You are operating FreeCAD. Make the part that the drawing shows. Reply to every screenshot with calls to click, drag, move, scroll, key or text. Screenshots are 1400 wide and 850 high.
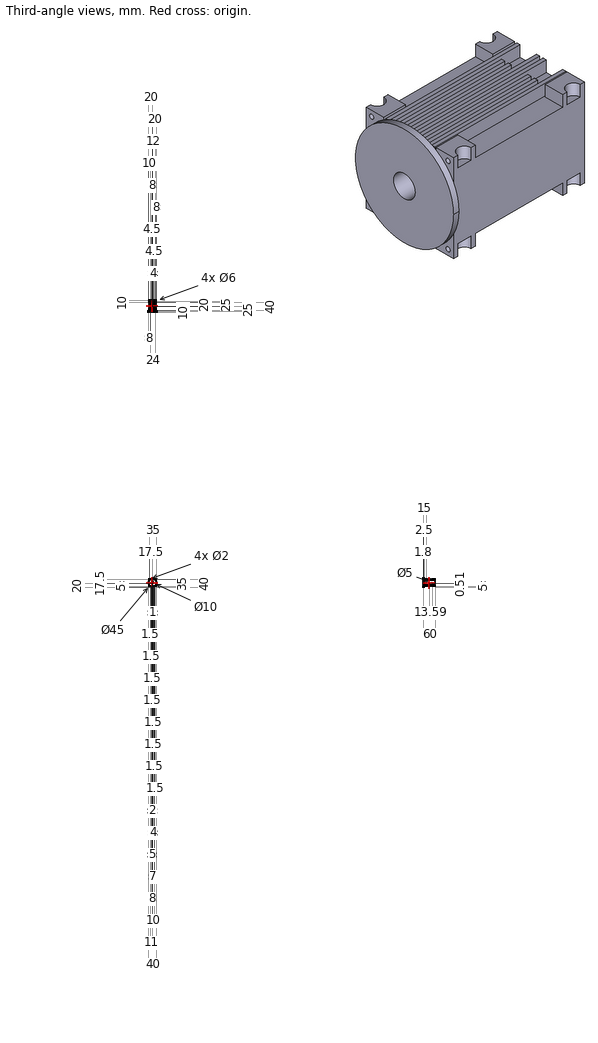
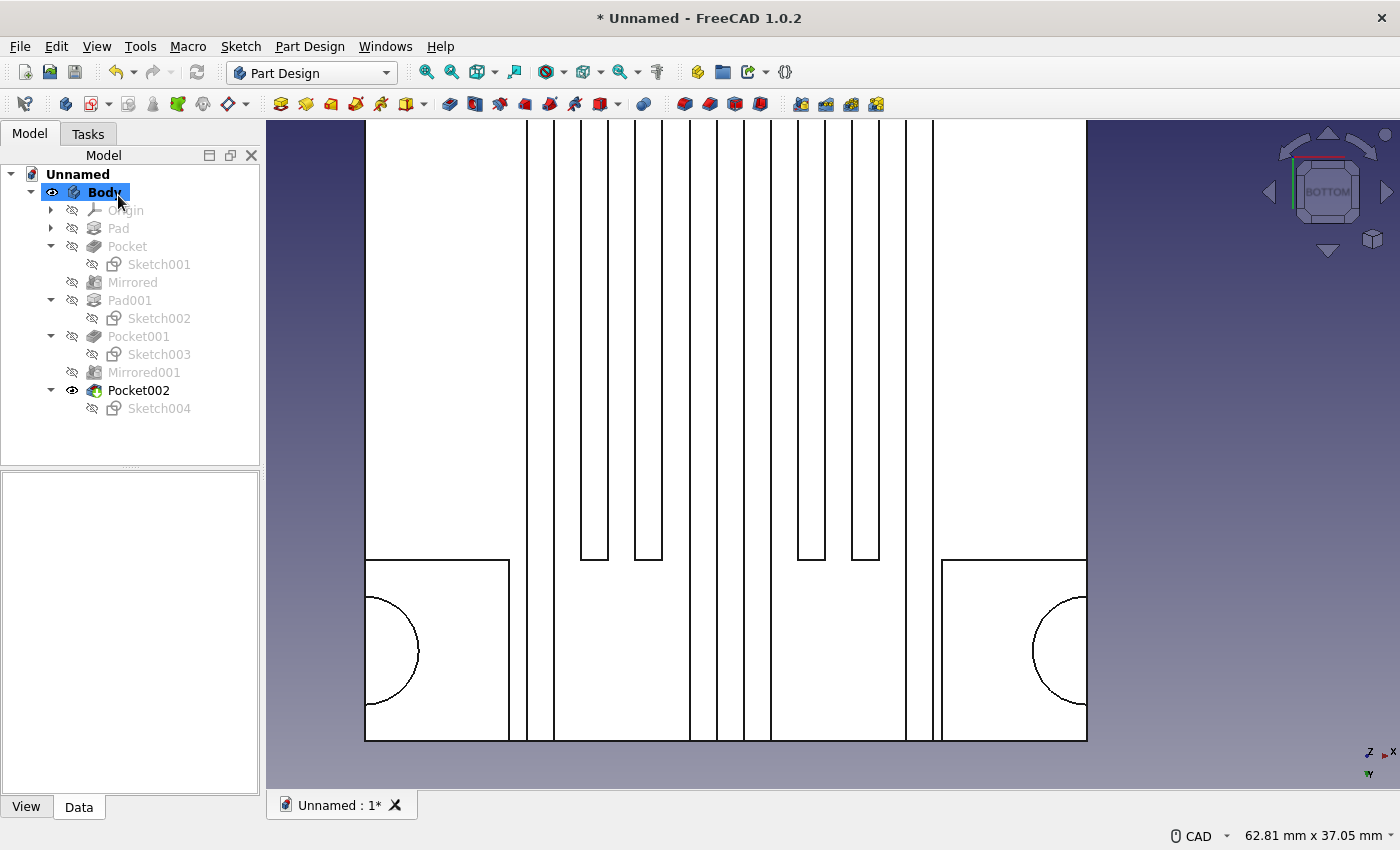
click(427, 72)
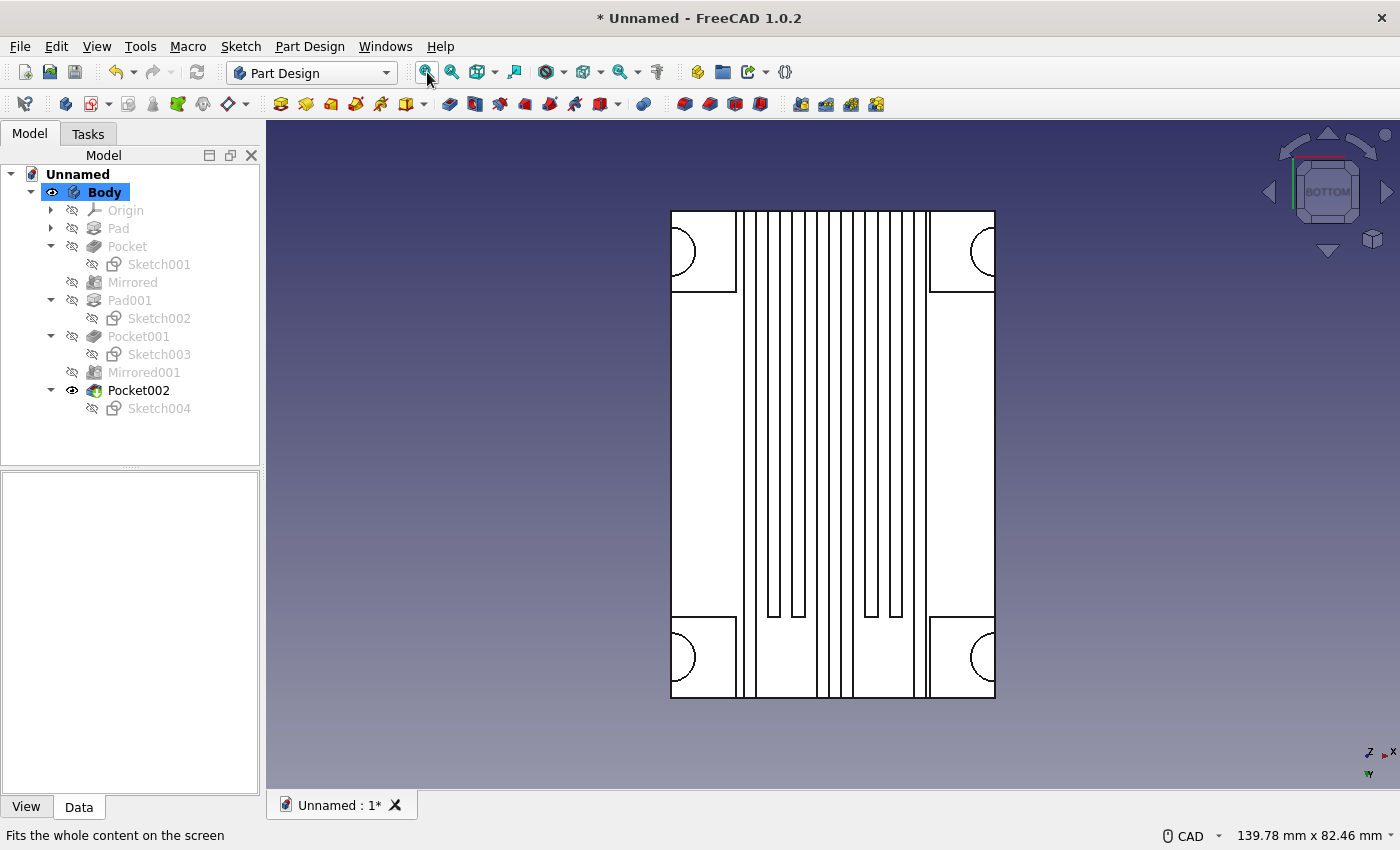
click(117, 390)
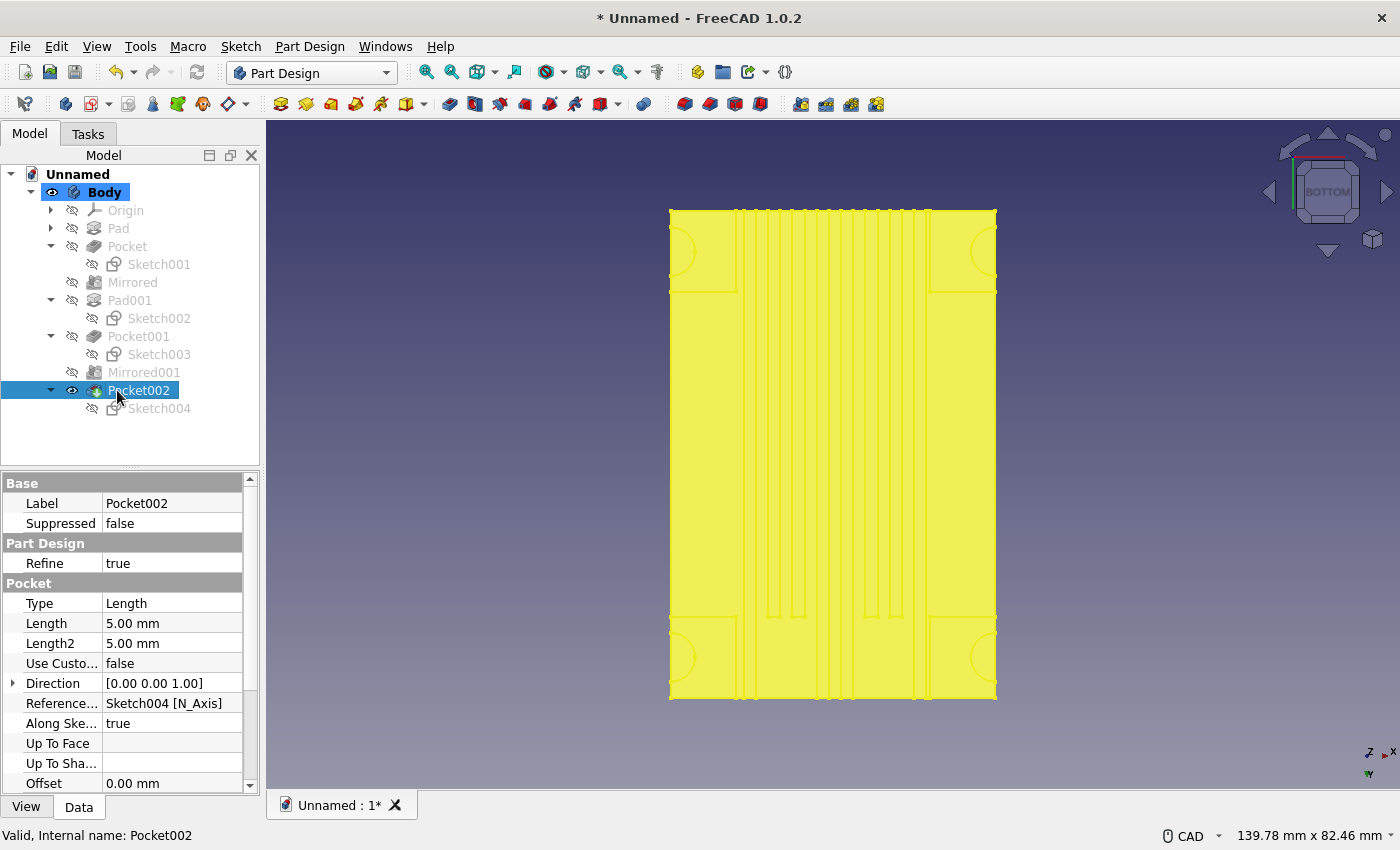
click(801, 104)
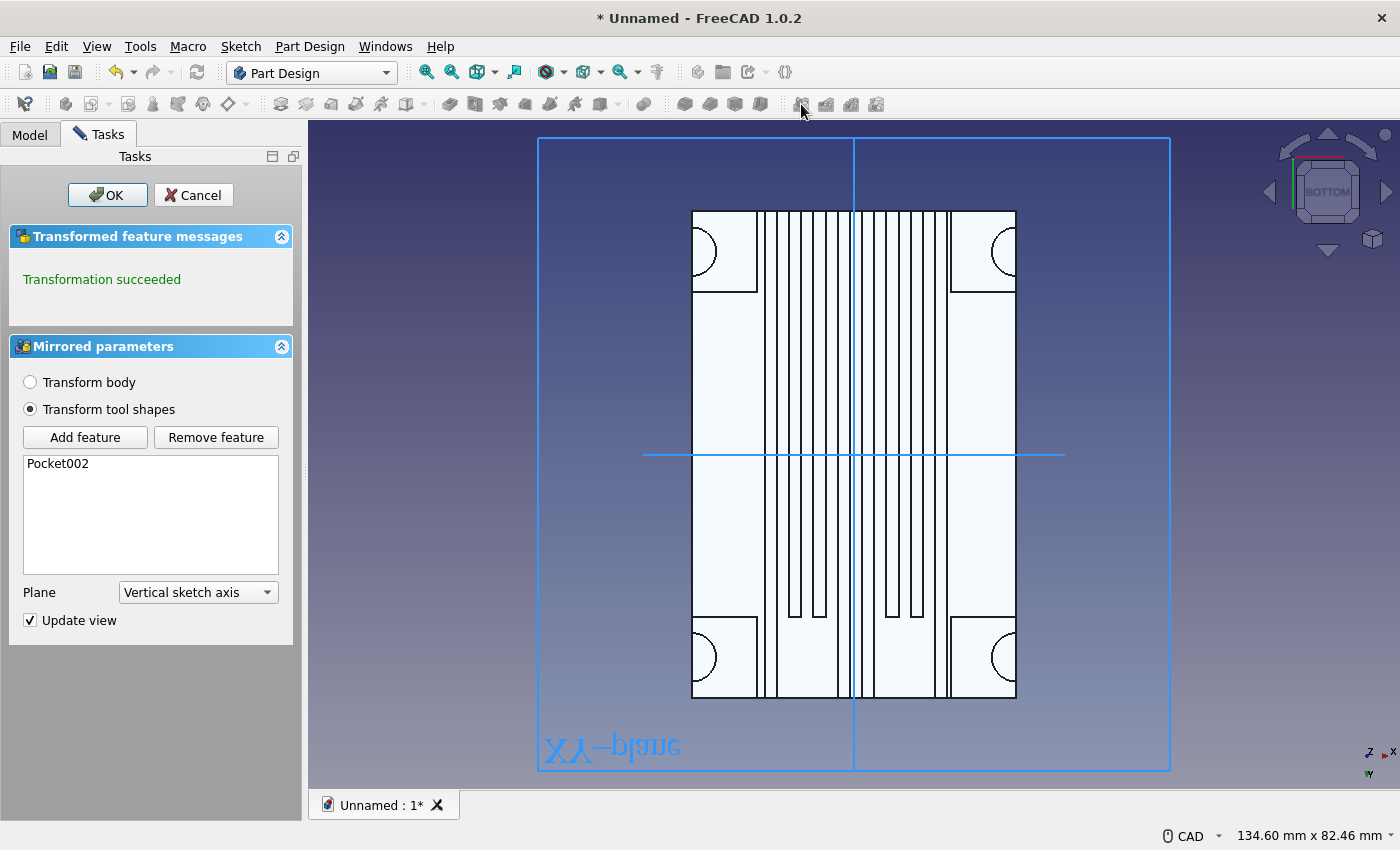
click(199, 592)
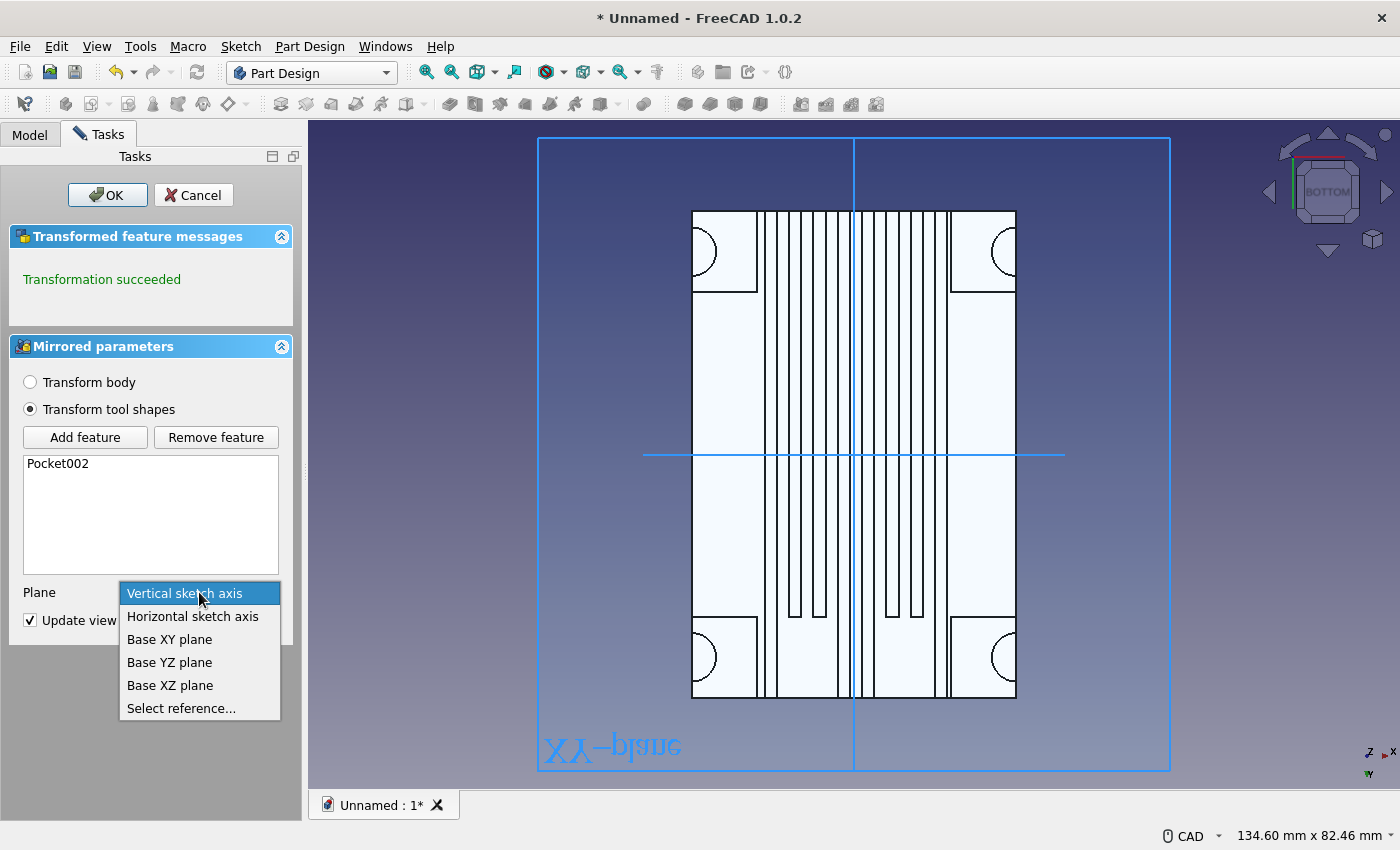
click(198, 640)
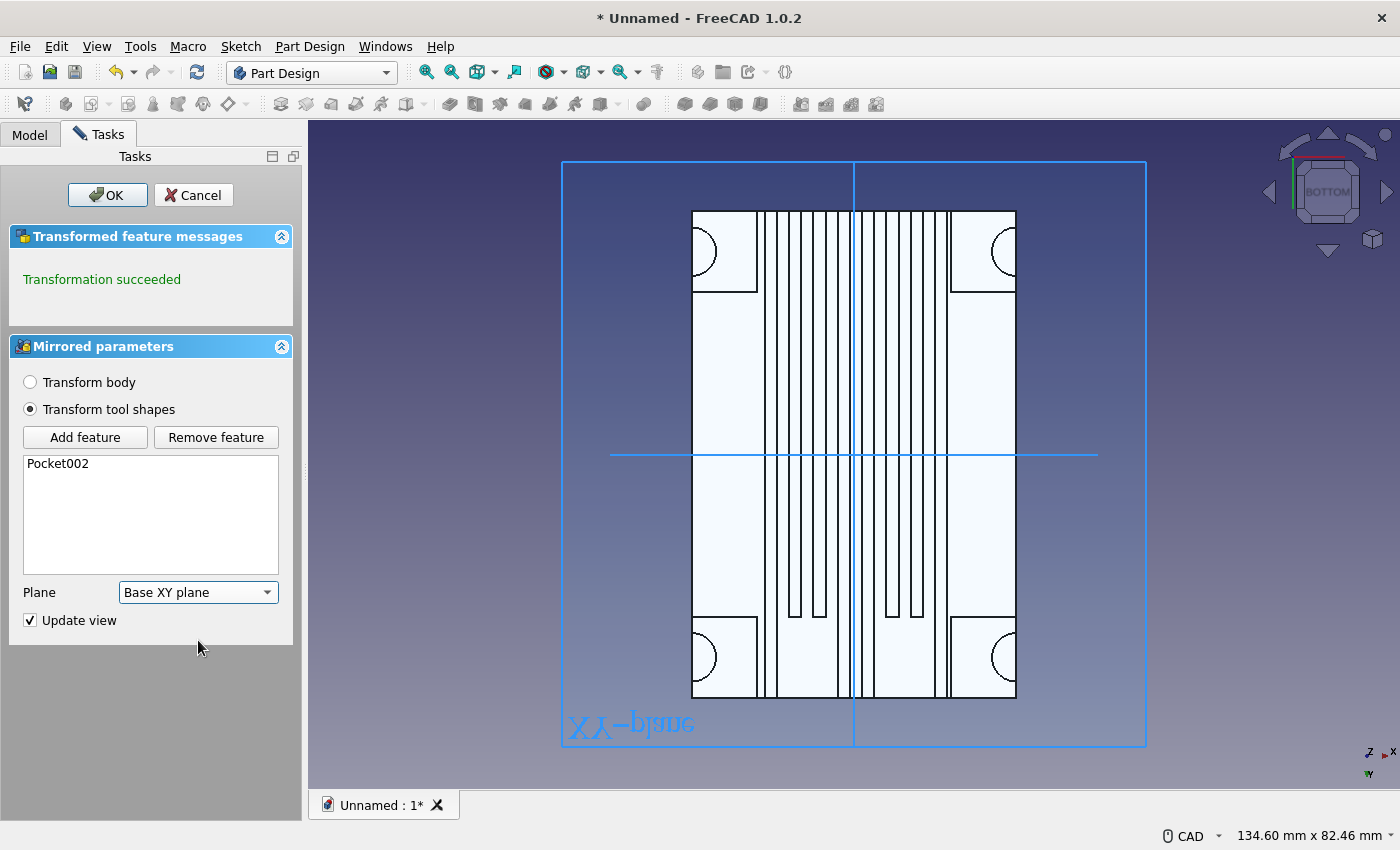
click(108, 195)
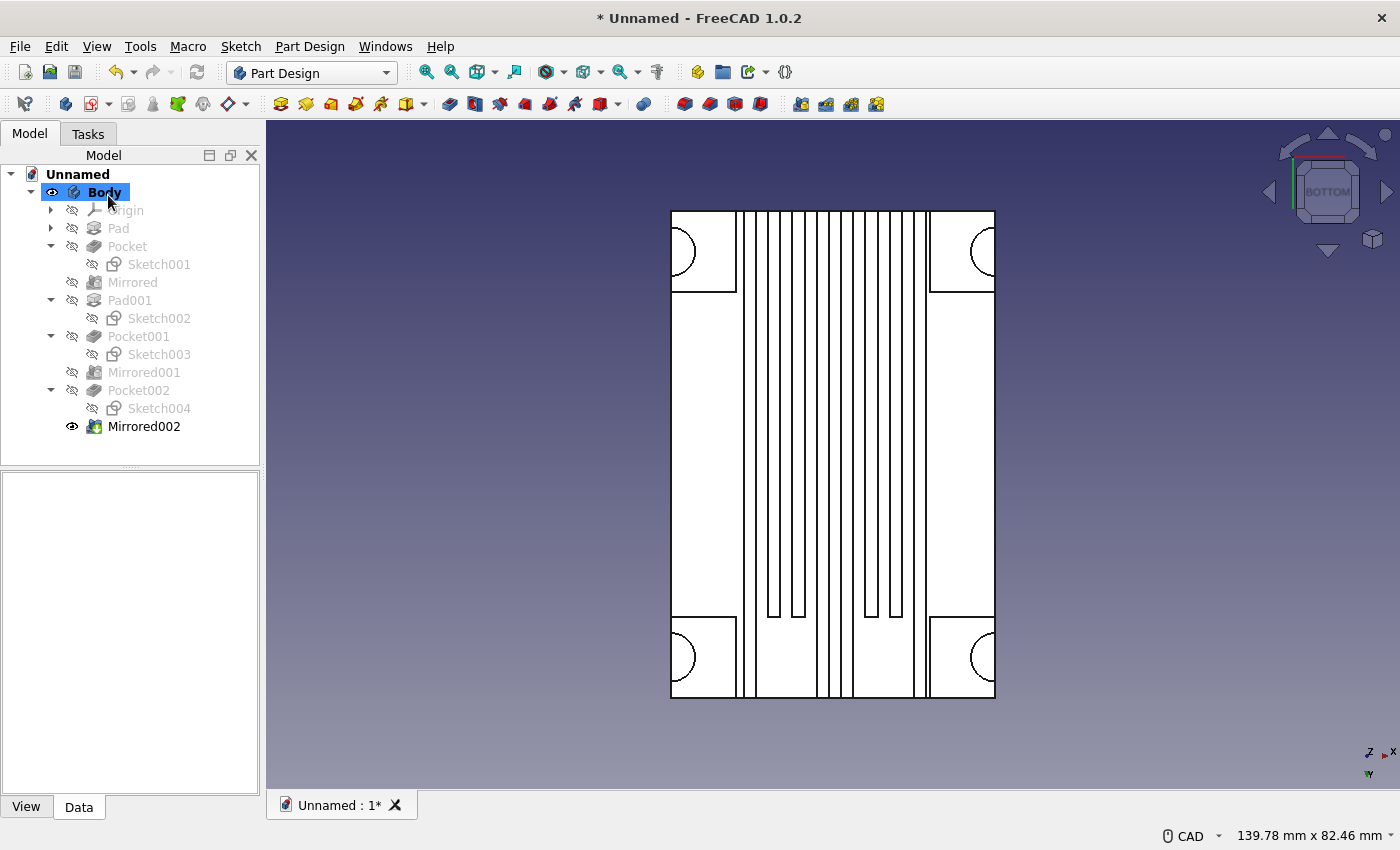
key(0)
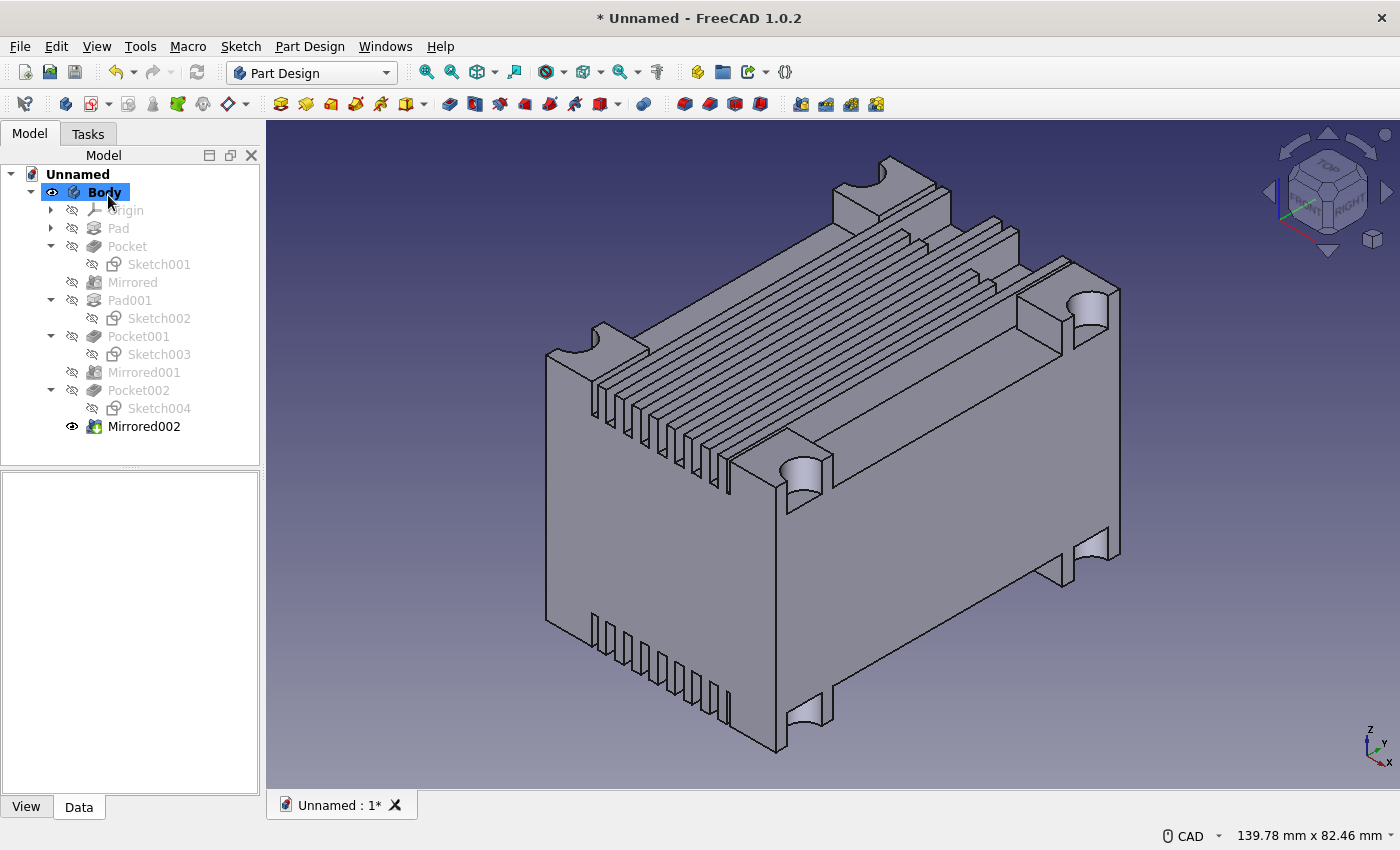
click(661, 553)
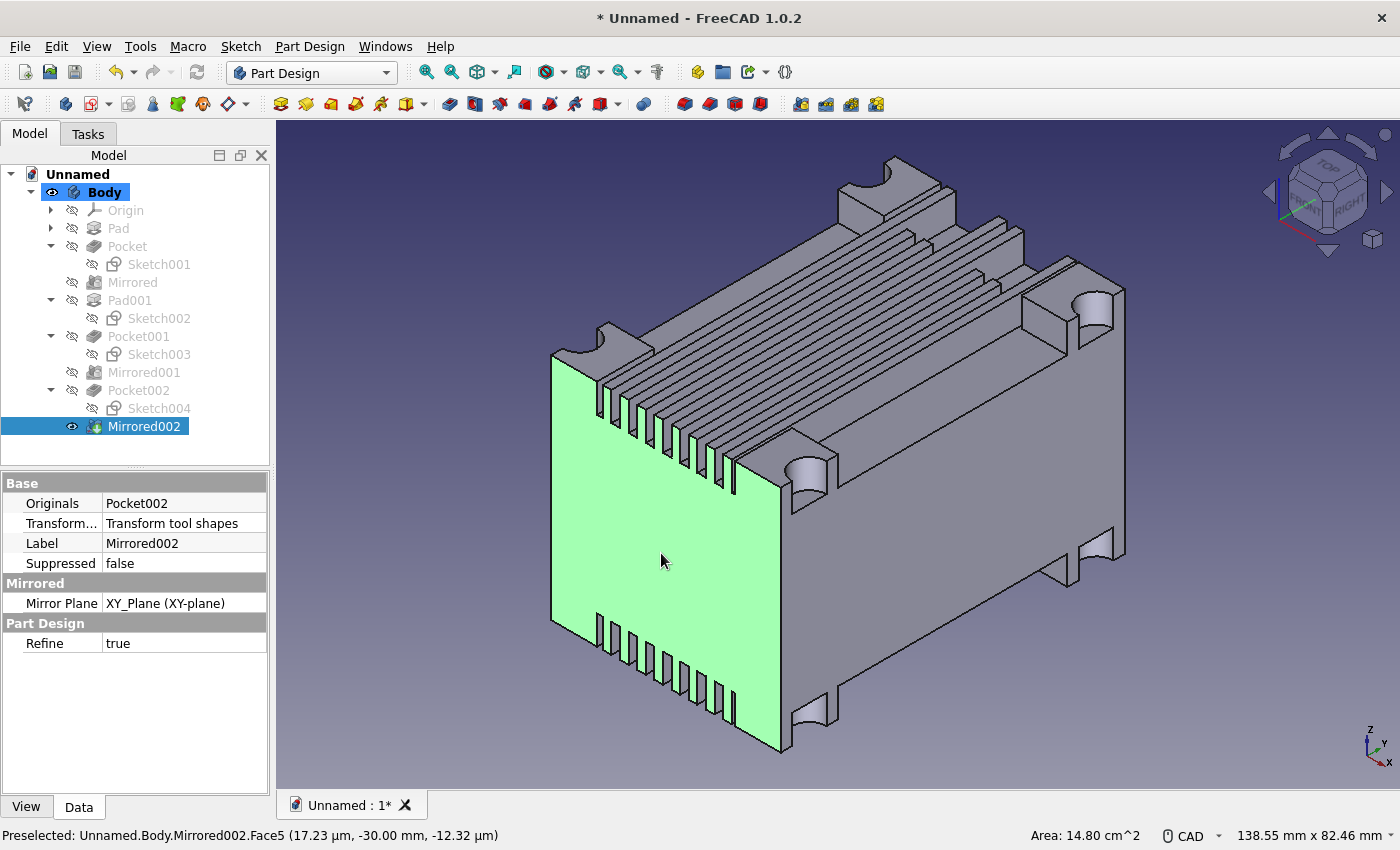
click(90, 104)